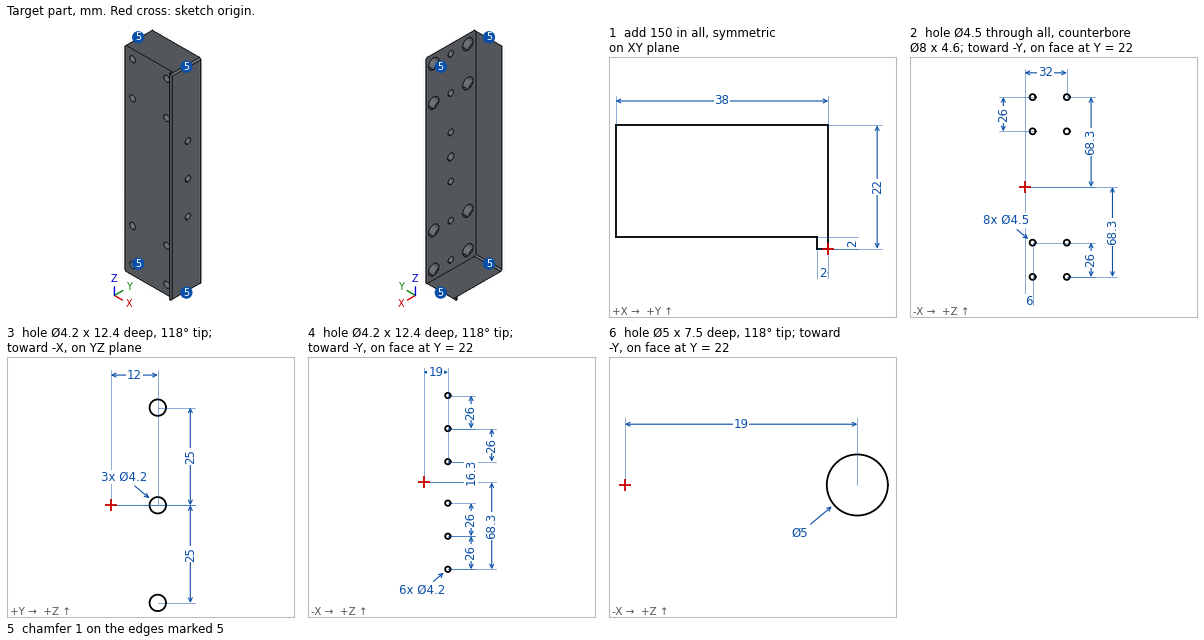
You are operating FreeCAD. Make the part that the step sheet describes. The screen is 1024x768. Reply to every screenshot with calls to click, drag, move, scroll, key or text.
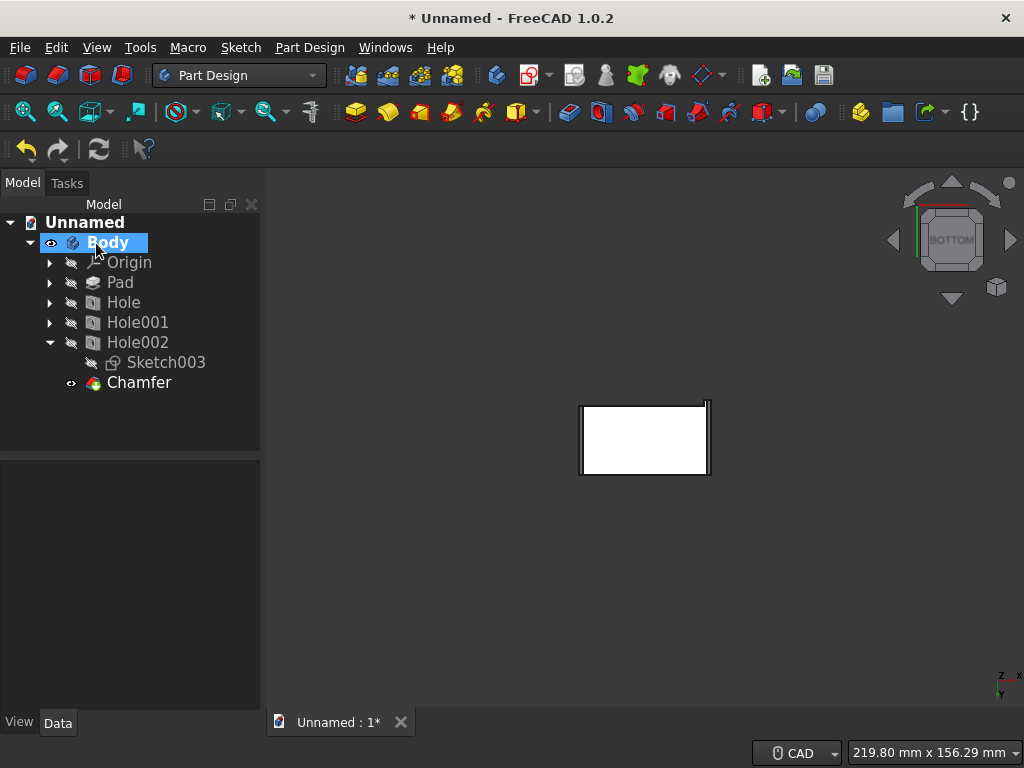
key(v)
key(f)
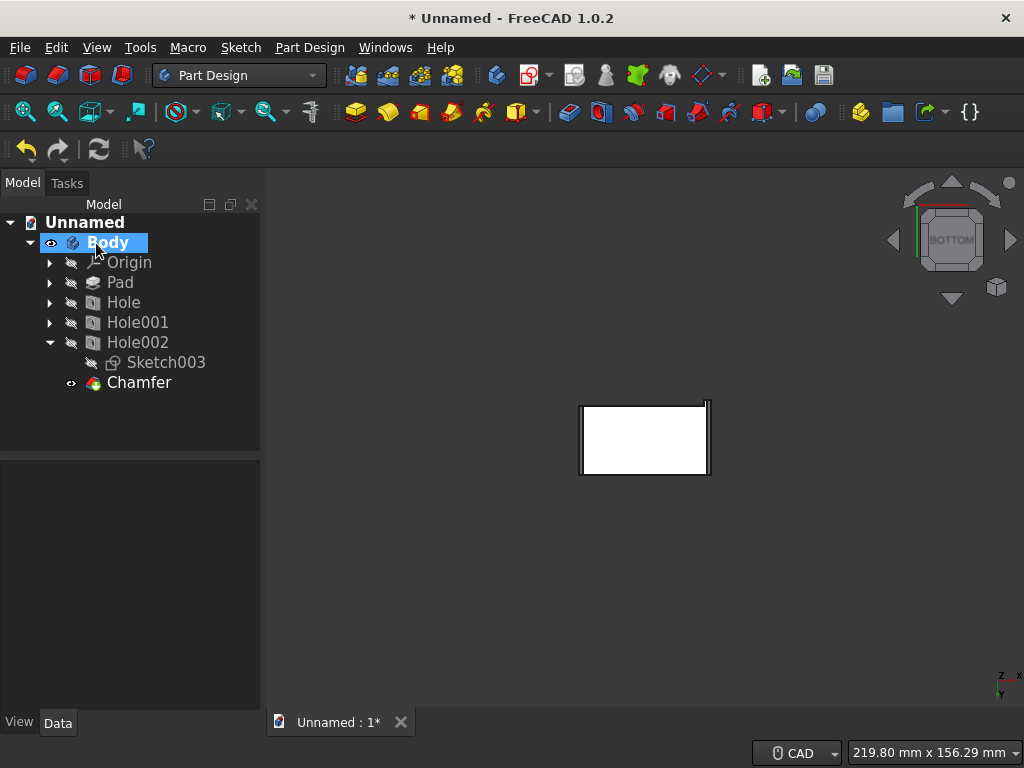
key(4)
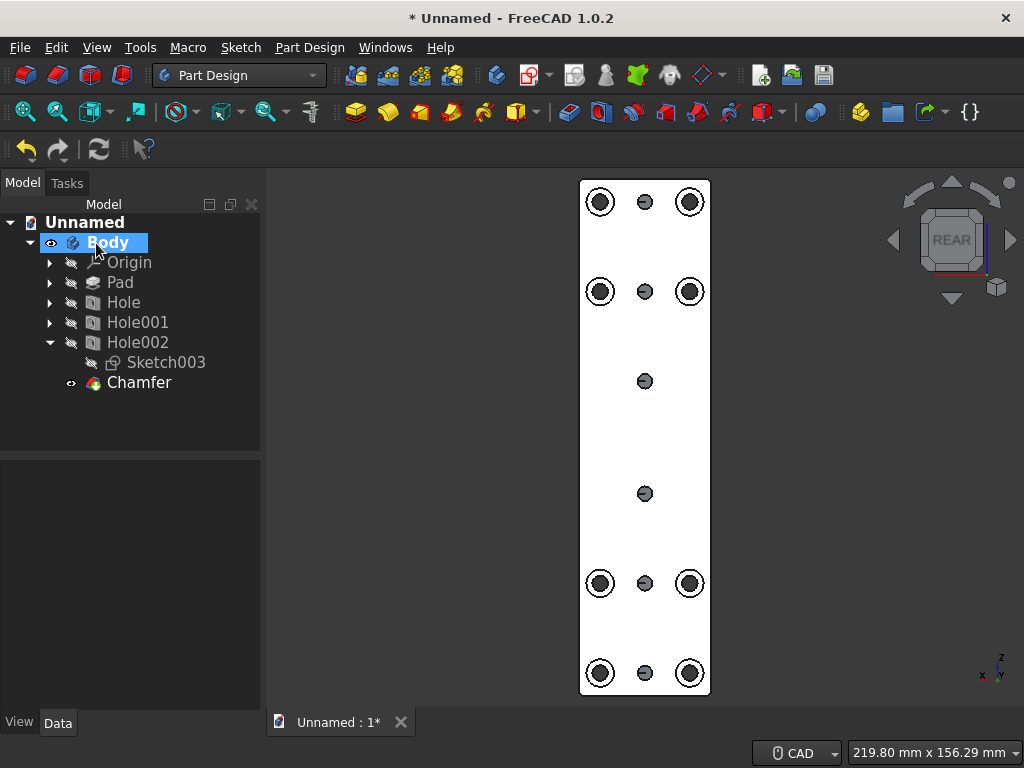
click(645, 436)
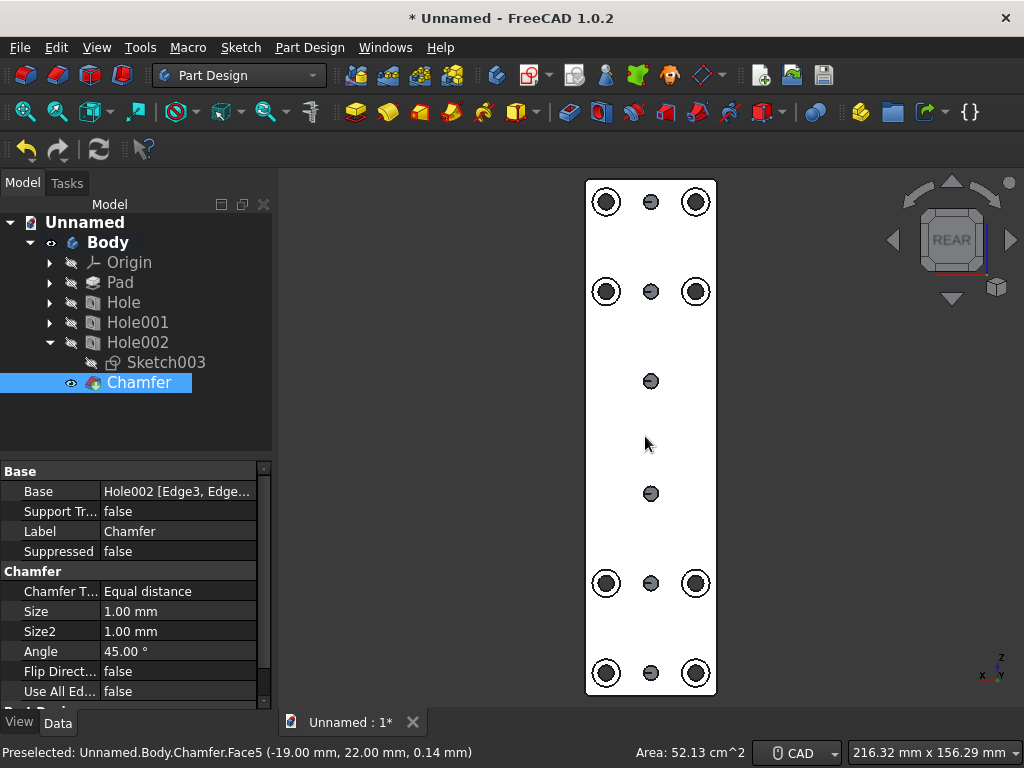
click(530, 76)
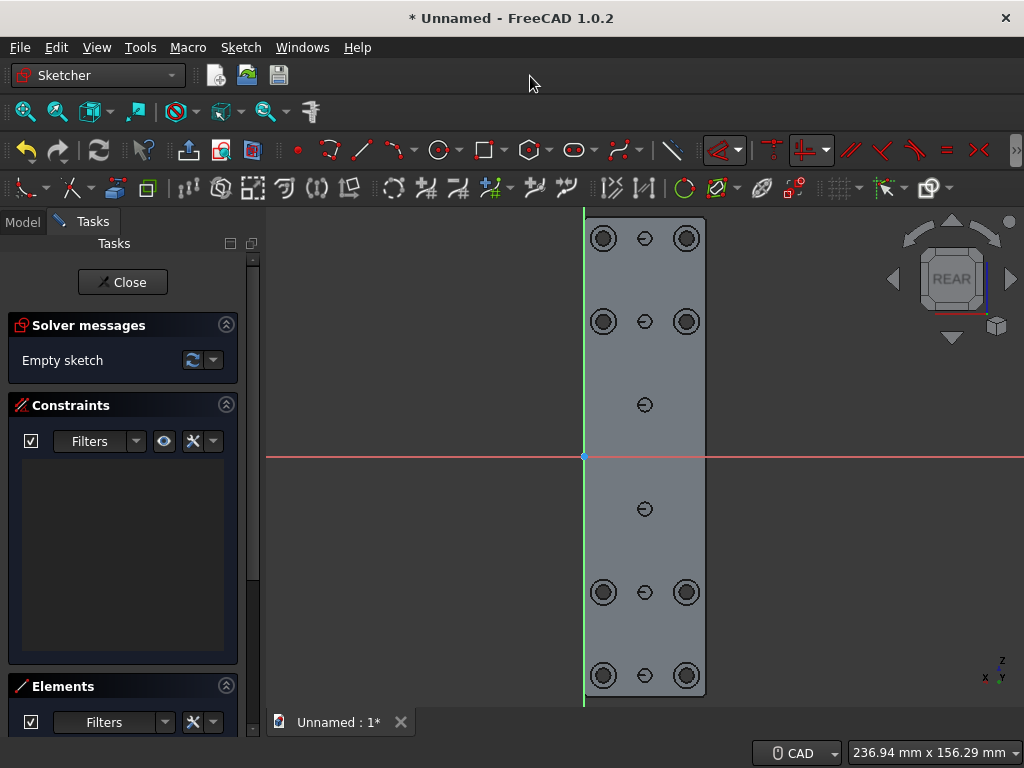
scroll(649, 457, up, 15)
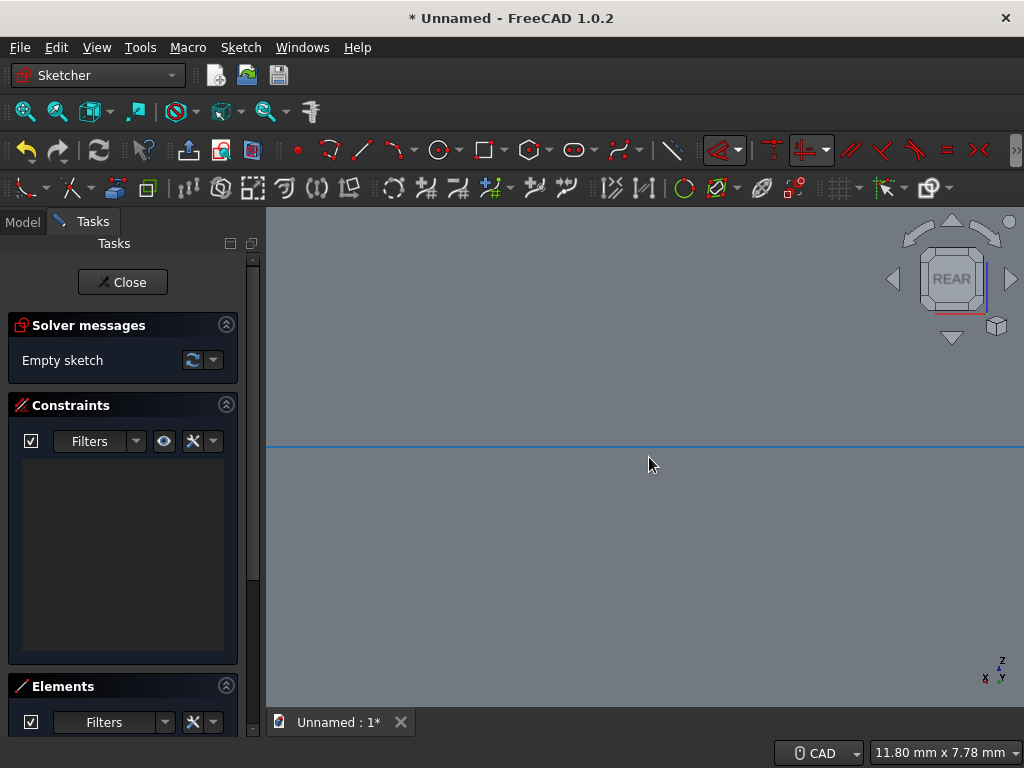
key(g)
key(c)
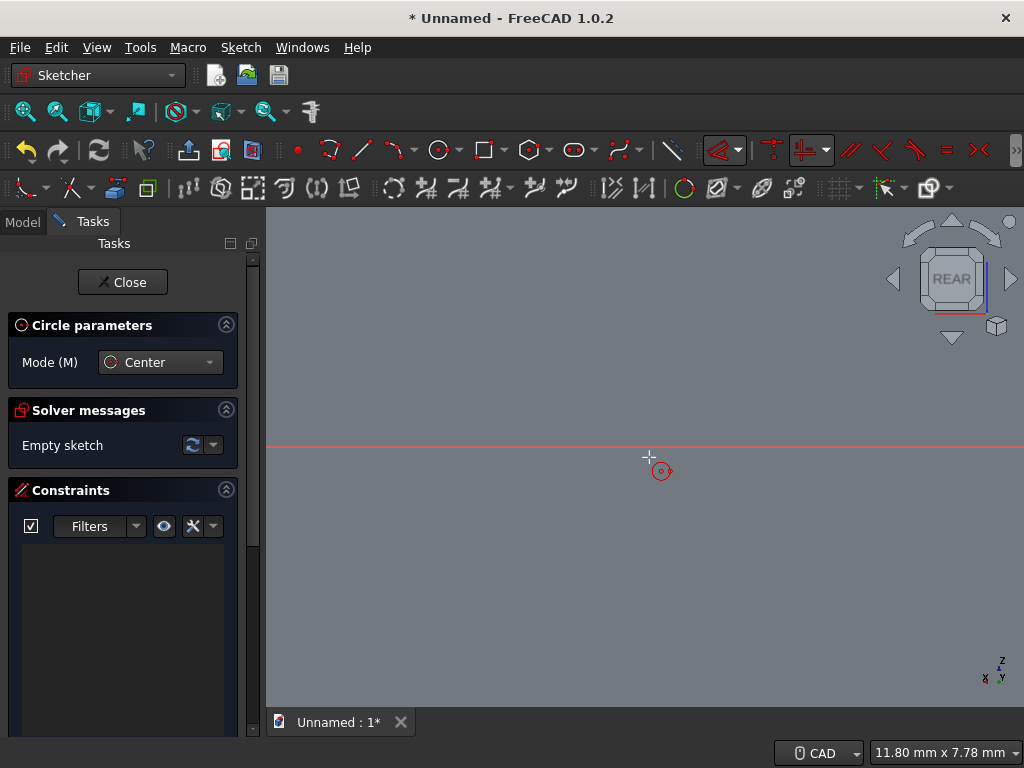
click(559, 447)
click(673, 334)
key(Escape)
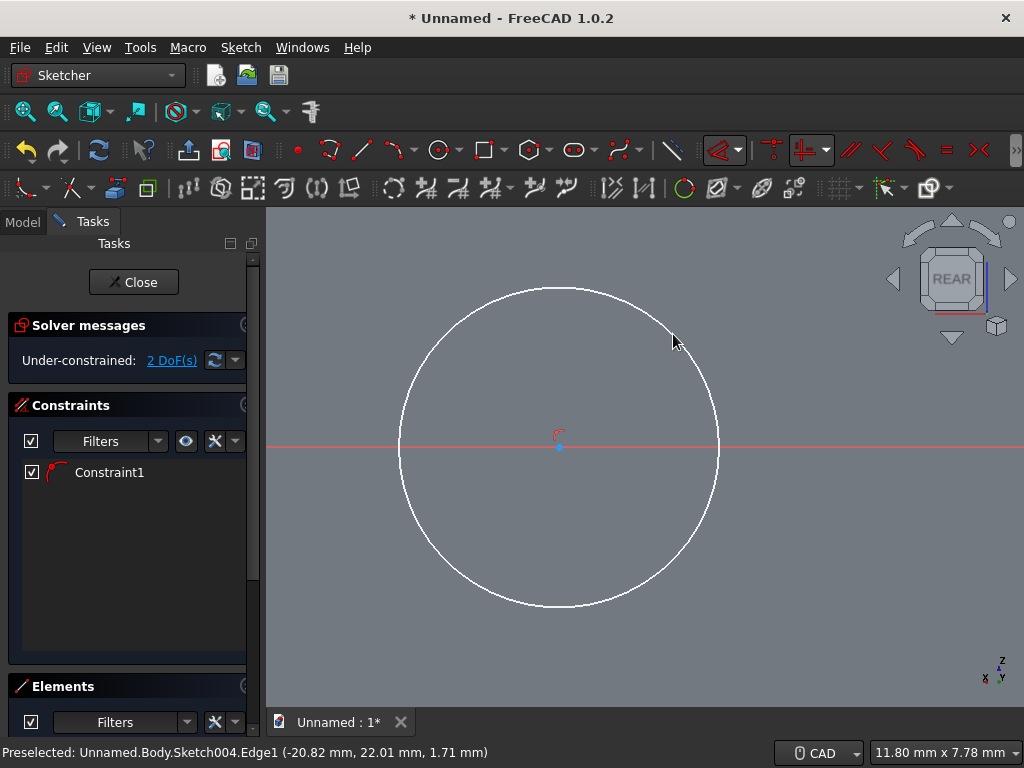
click(672, 334)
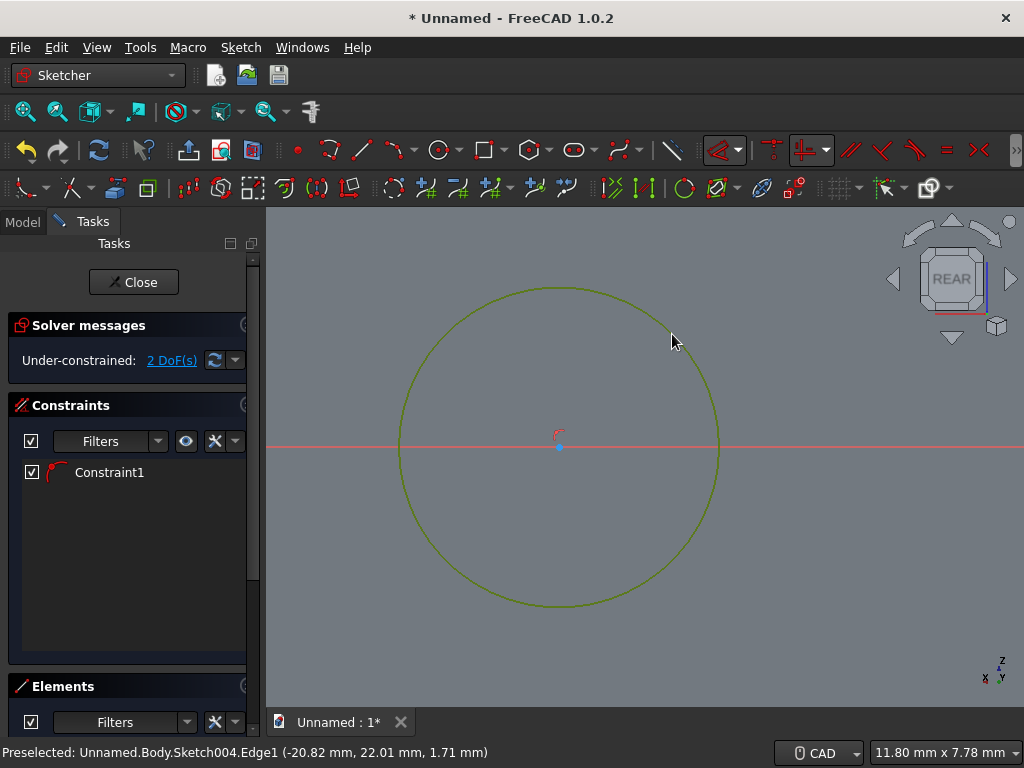
key(k)
key(o)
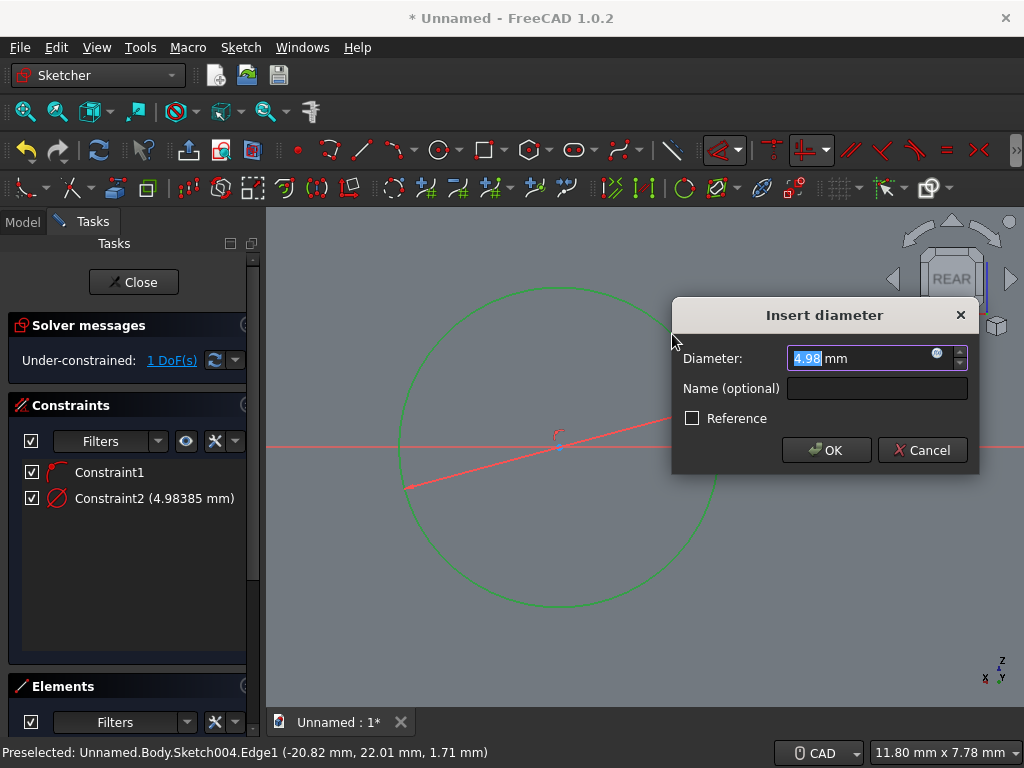
text(5)
key(Return)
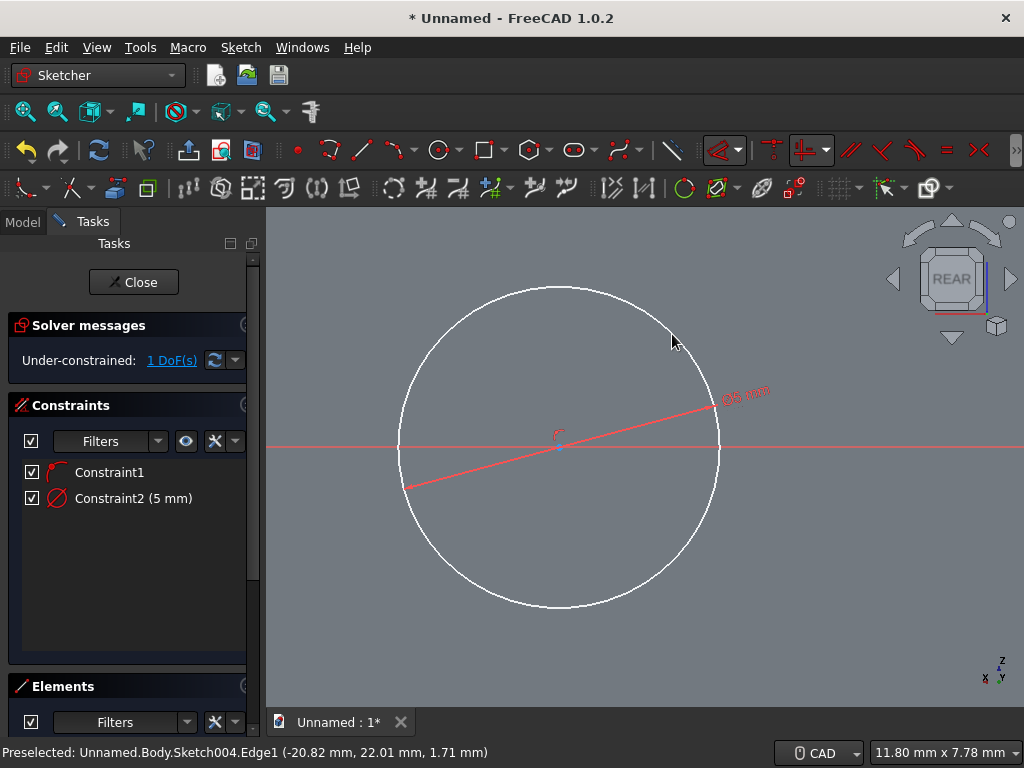
click(559, 447)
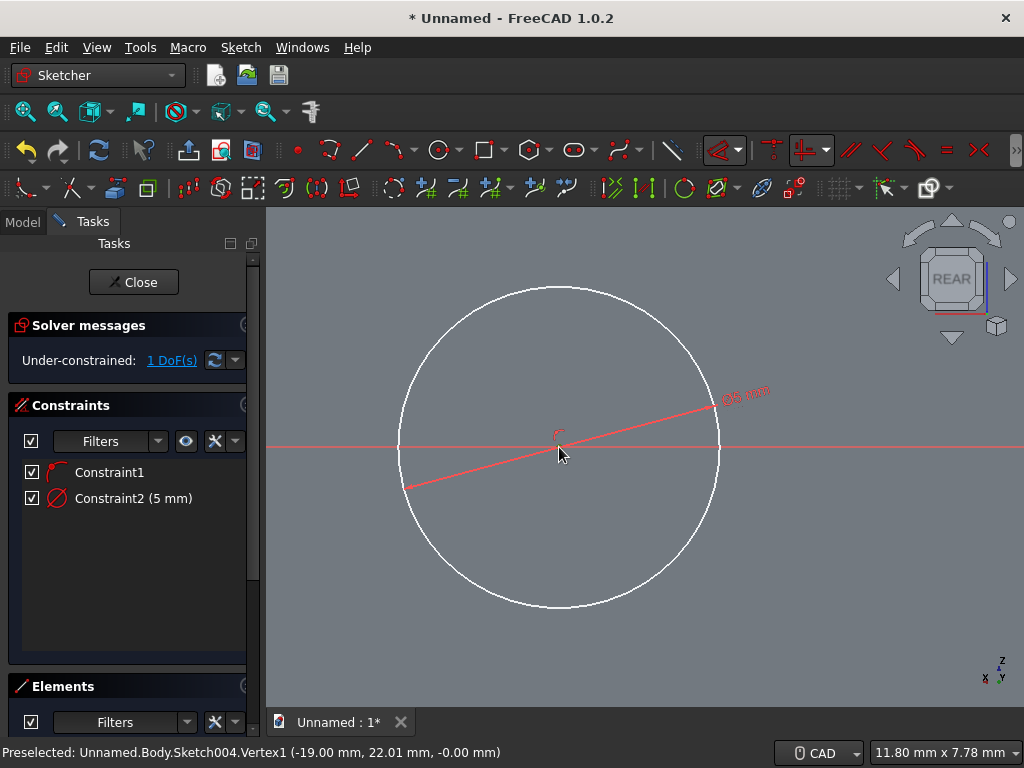
key(l)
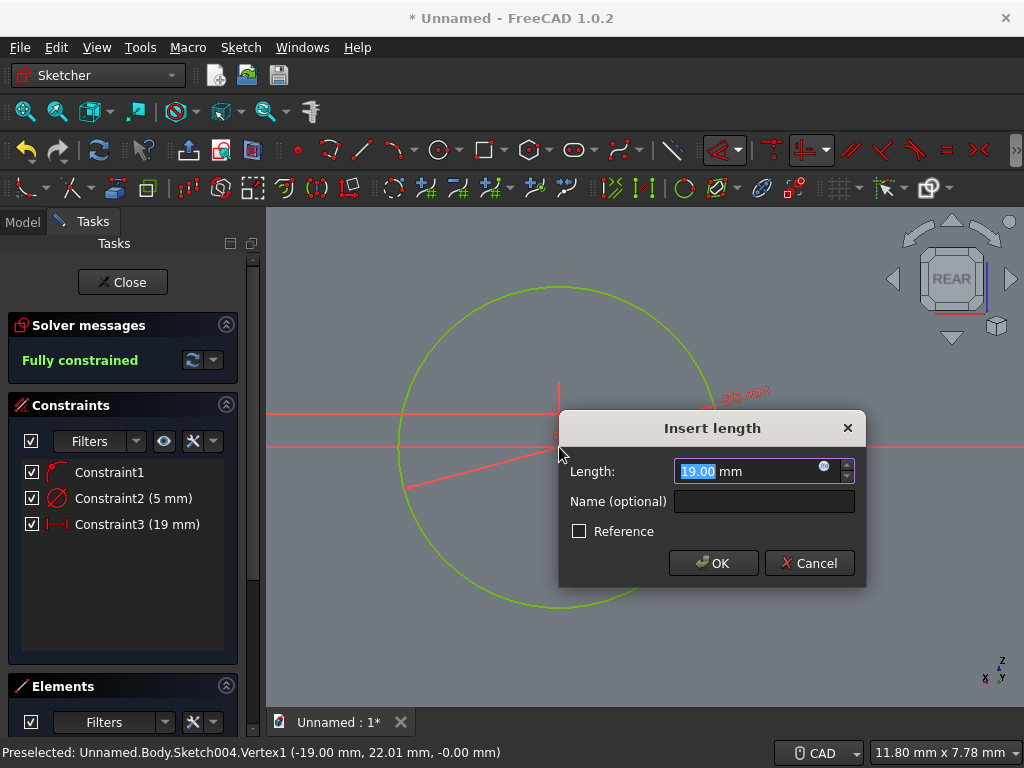
text(19)
key(Return)